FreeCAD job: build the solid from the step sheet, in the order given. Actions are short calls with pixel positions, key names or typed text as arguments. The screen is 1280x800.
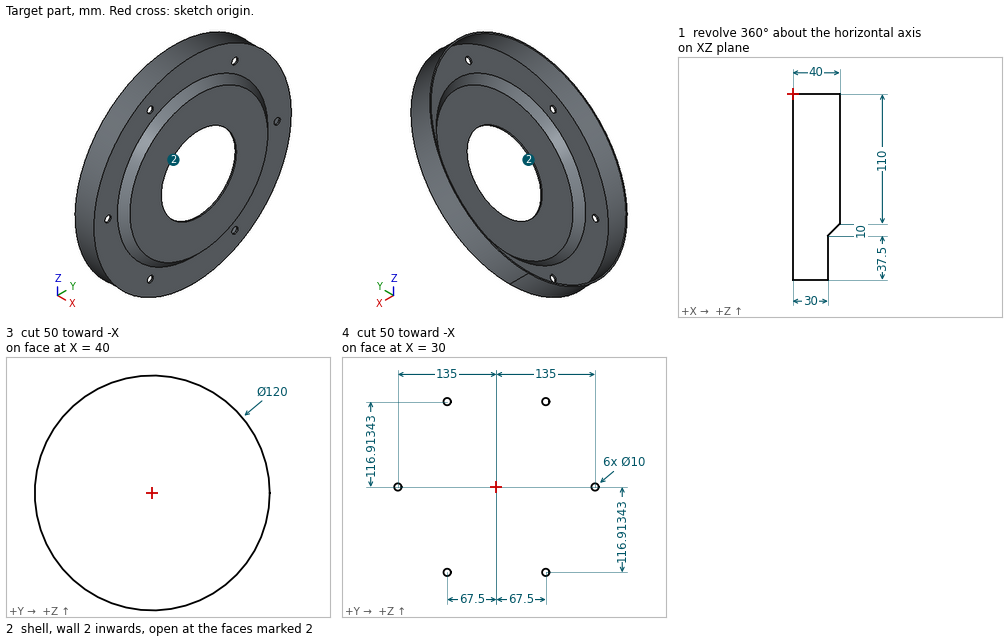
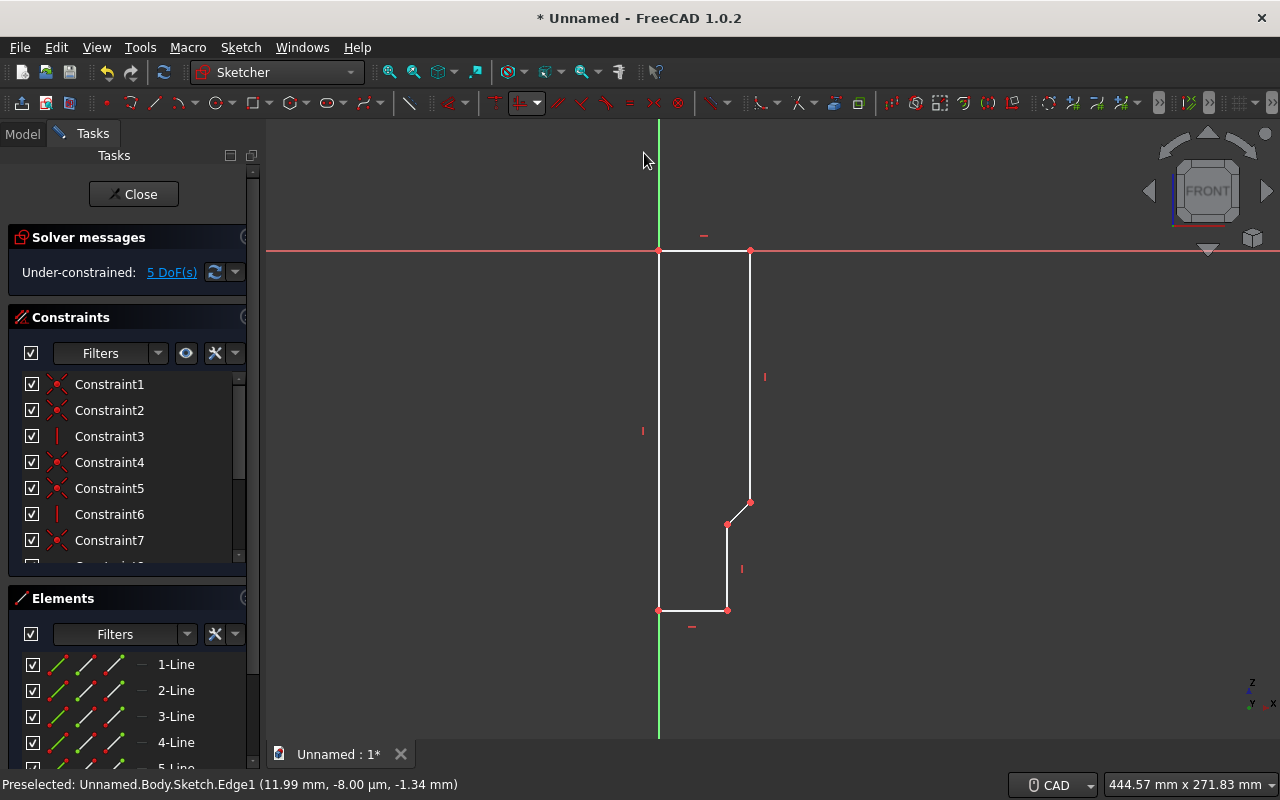
click(448, 104)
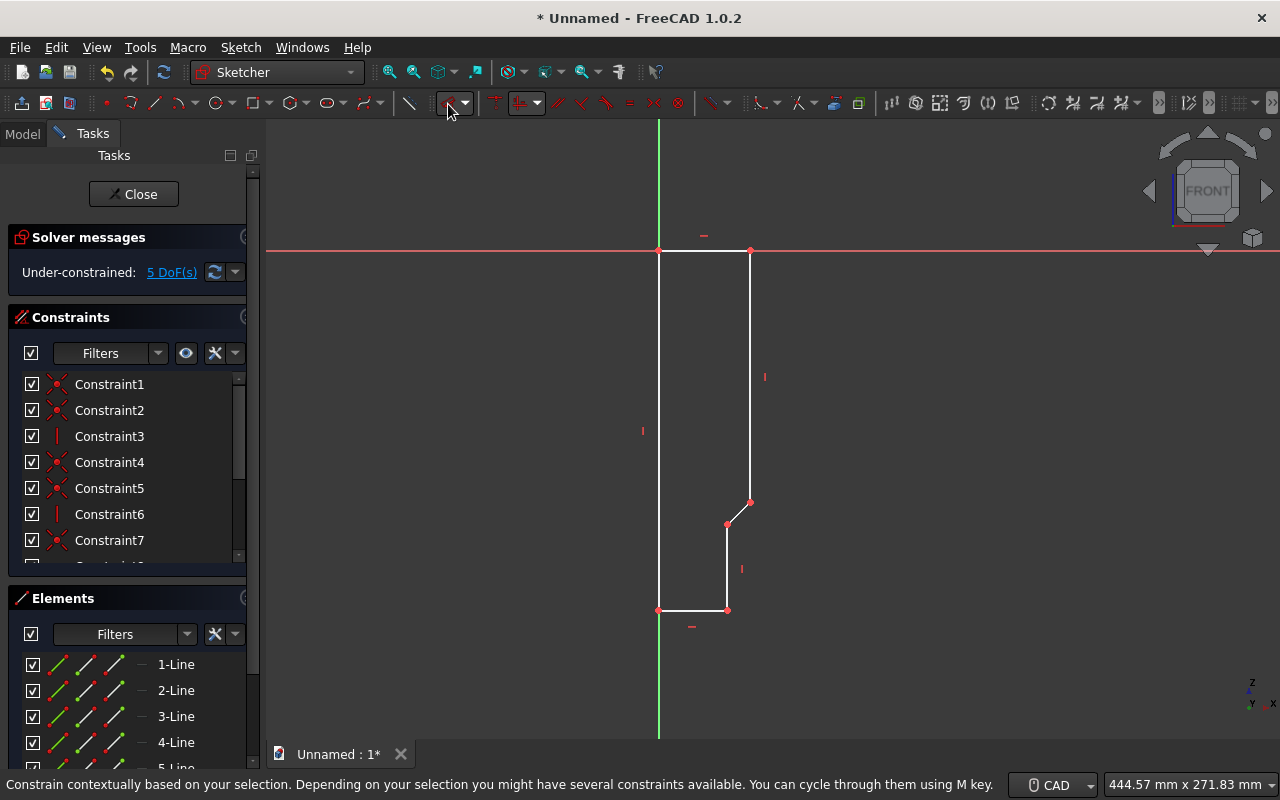
click(686, 251)
click(704, 217)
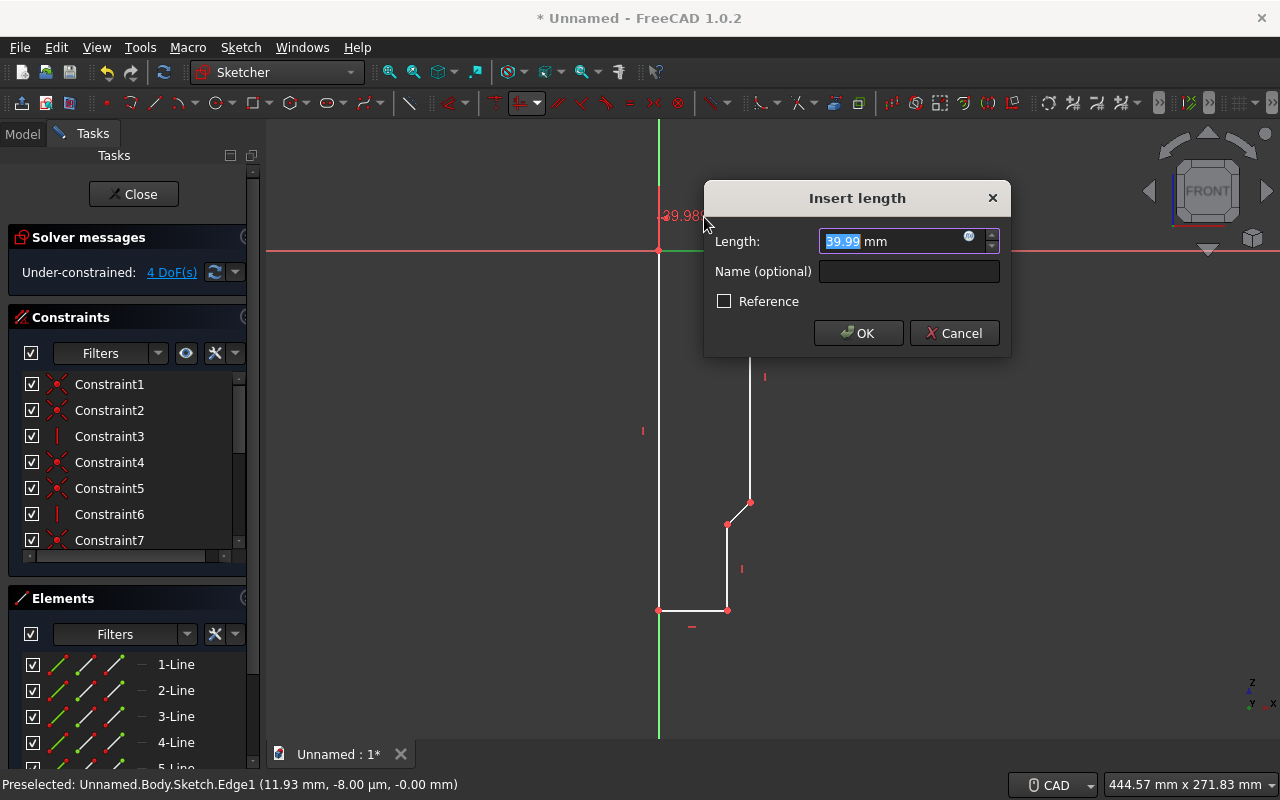
text(40)
key(Return)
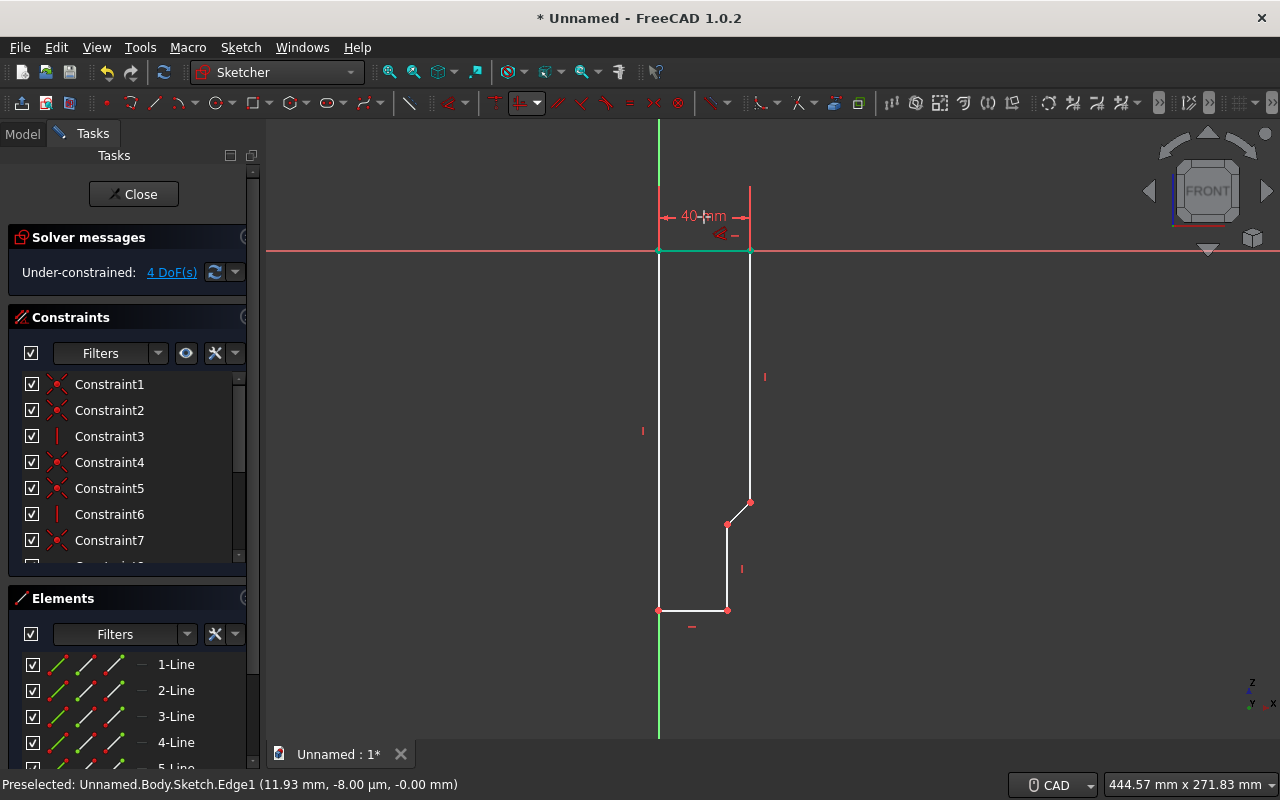
click(707, 611)
click(693, 645)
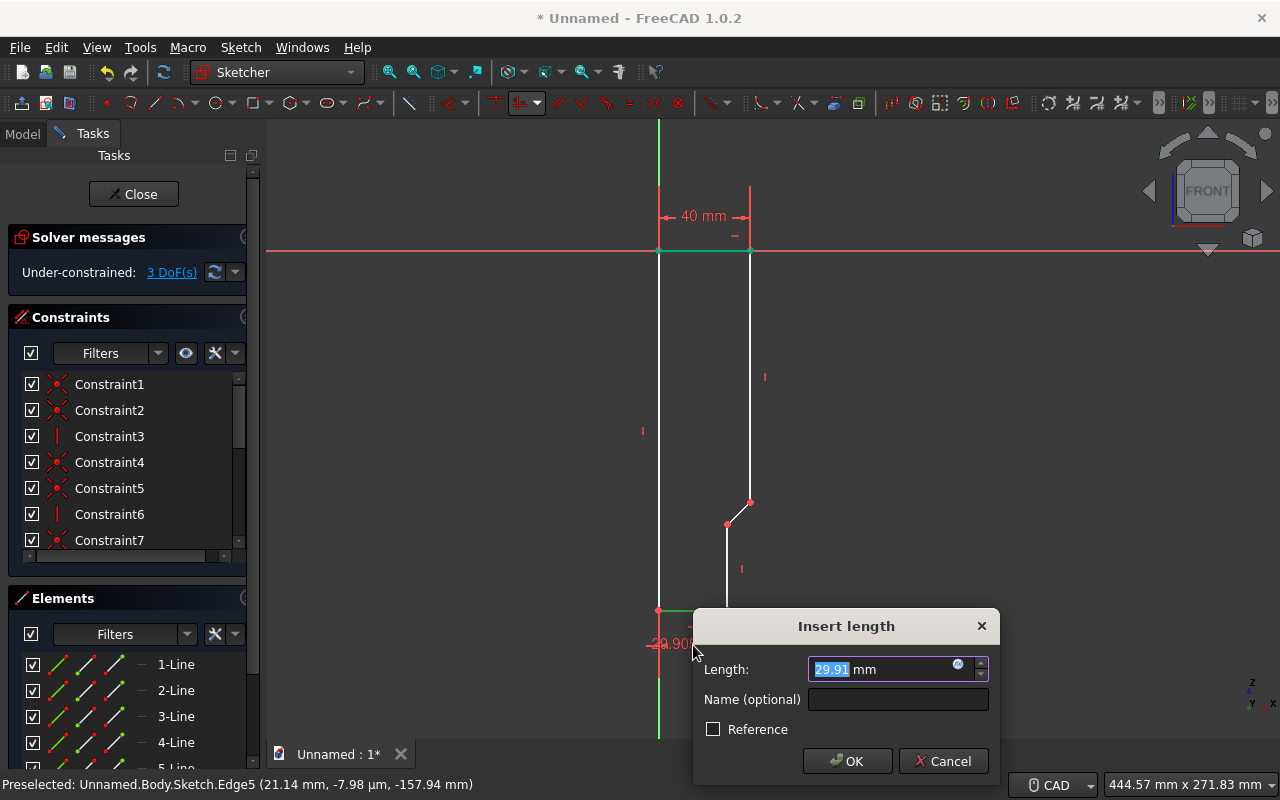
text(30)
key(Return)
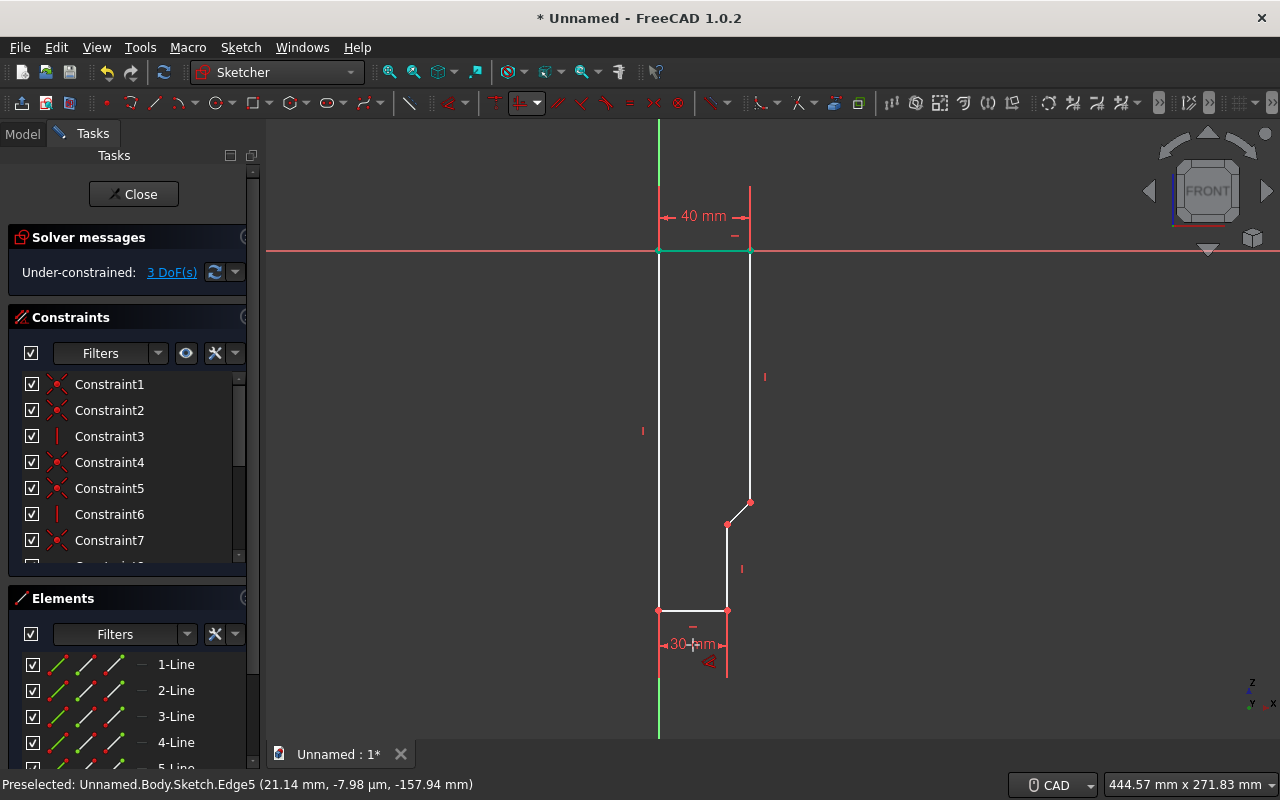
click(750, 326)
click(784, 377)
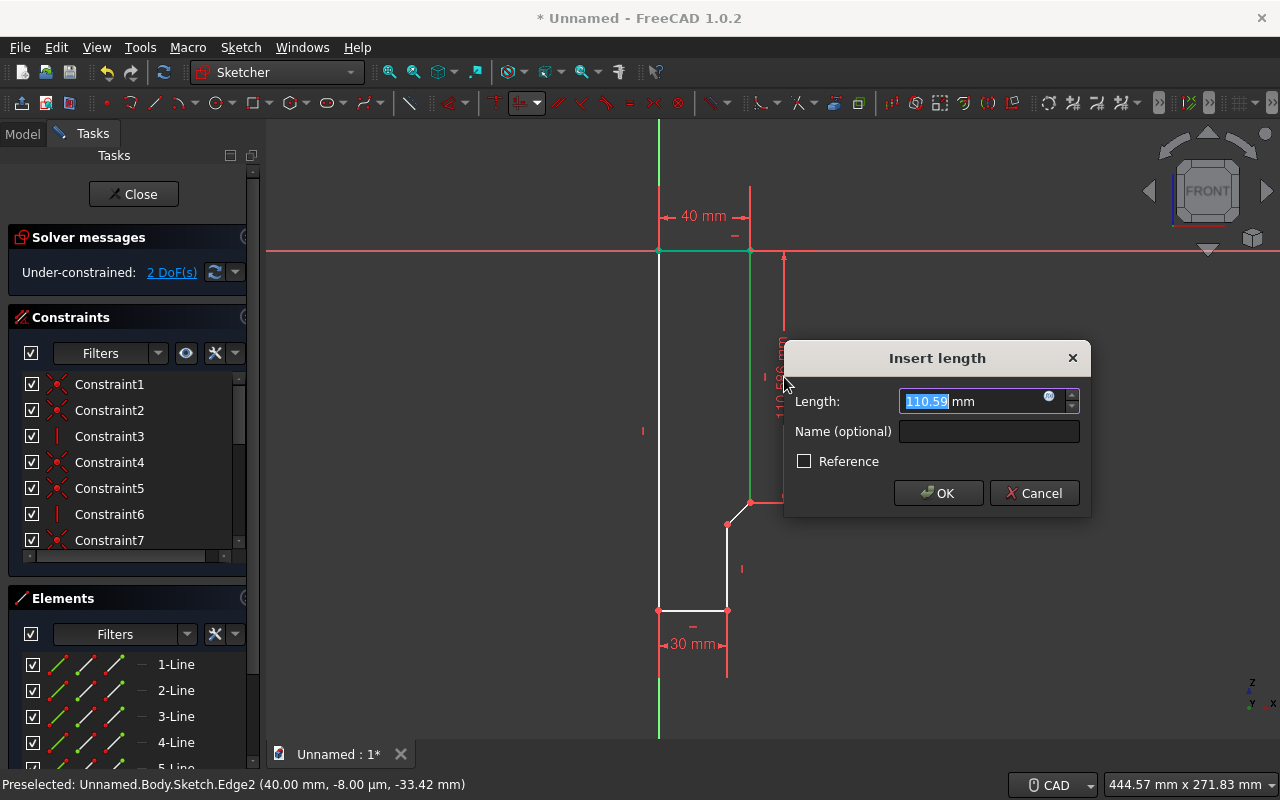
text(110)
key(Return)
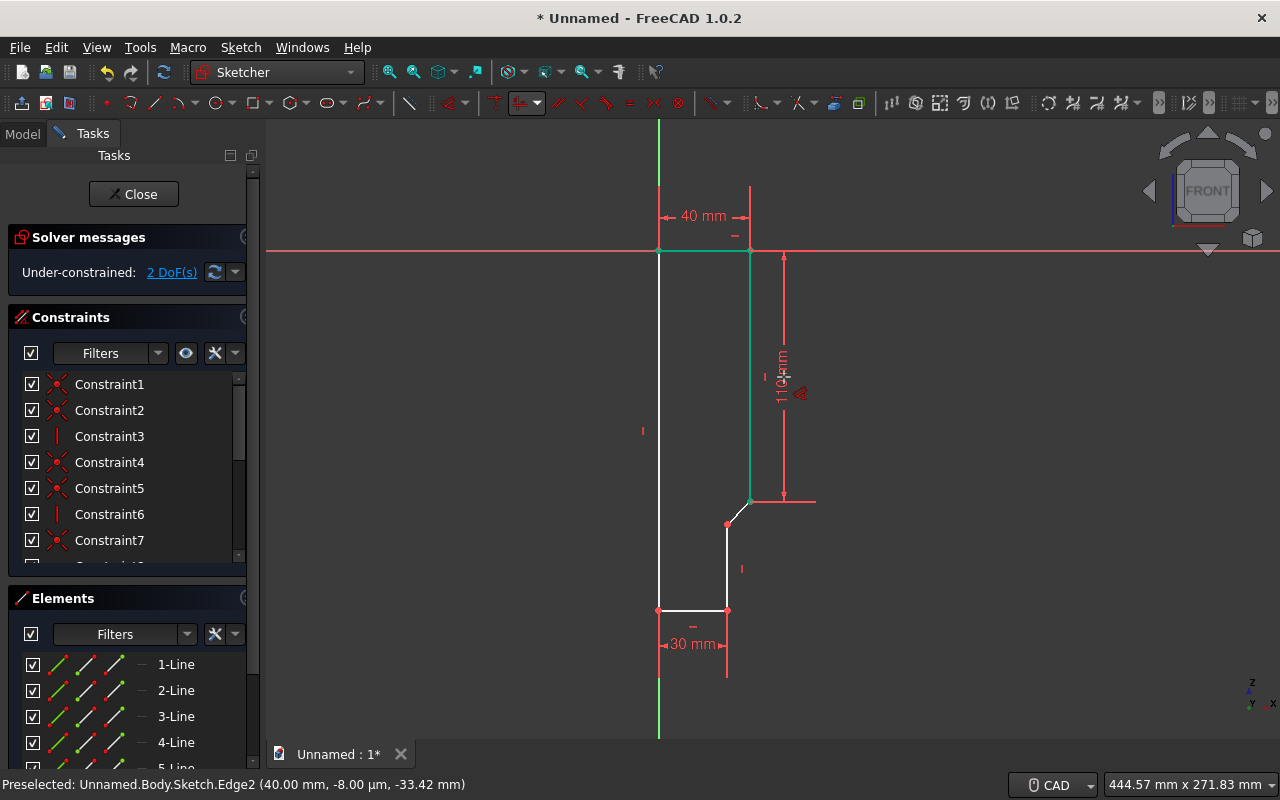
scroll(743, 509, up, 3)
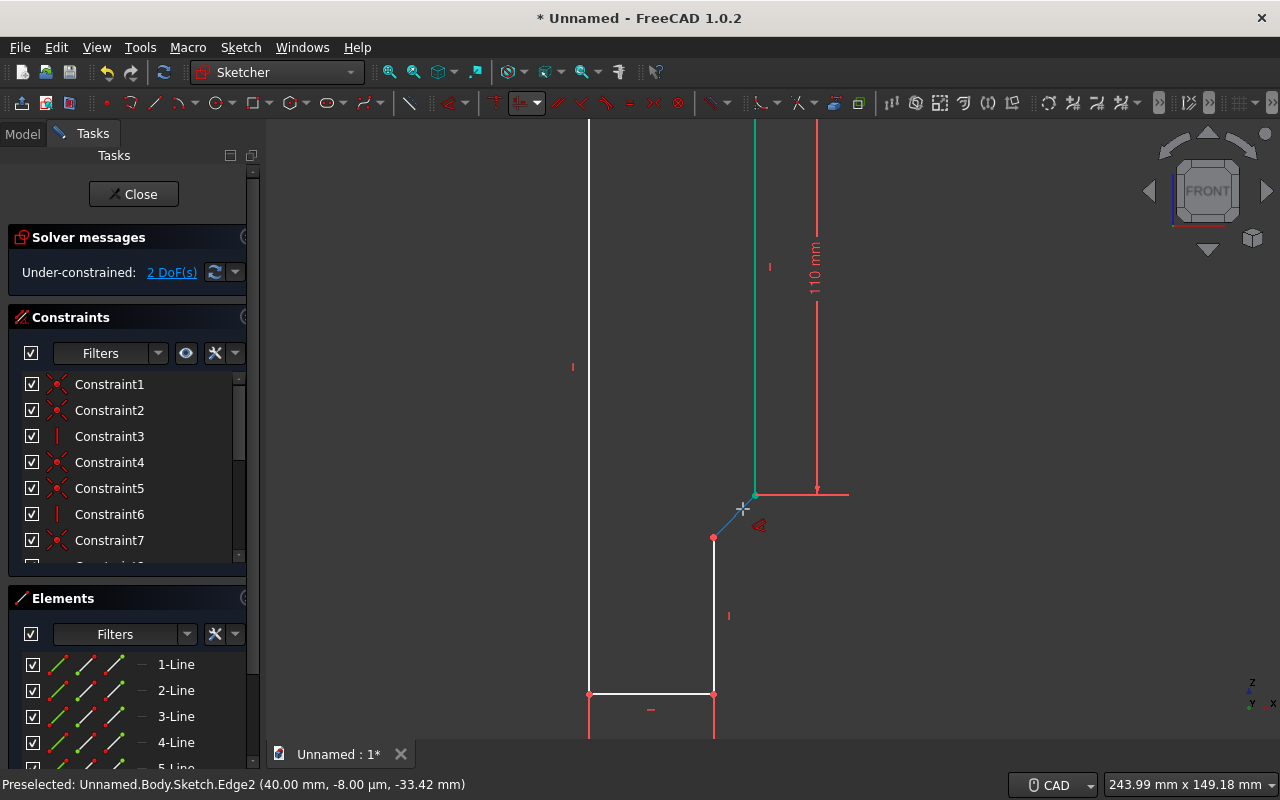
click(743, 508)
click(789, 516)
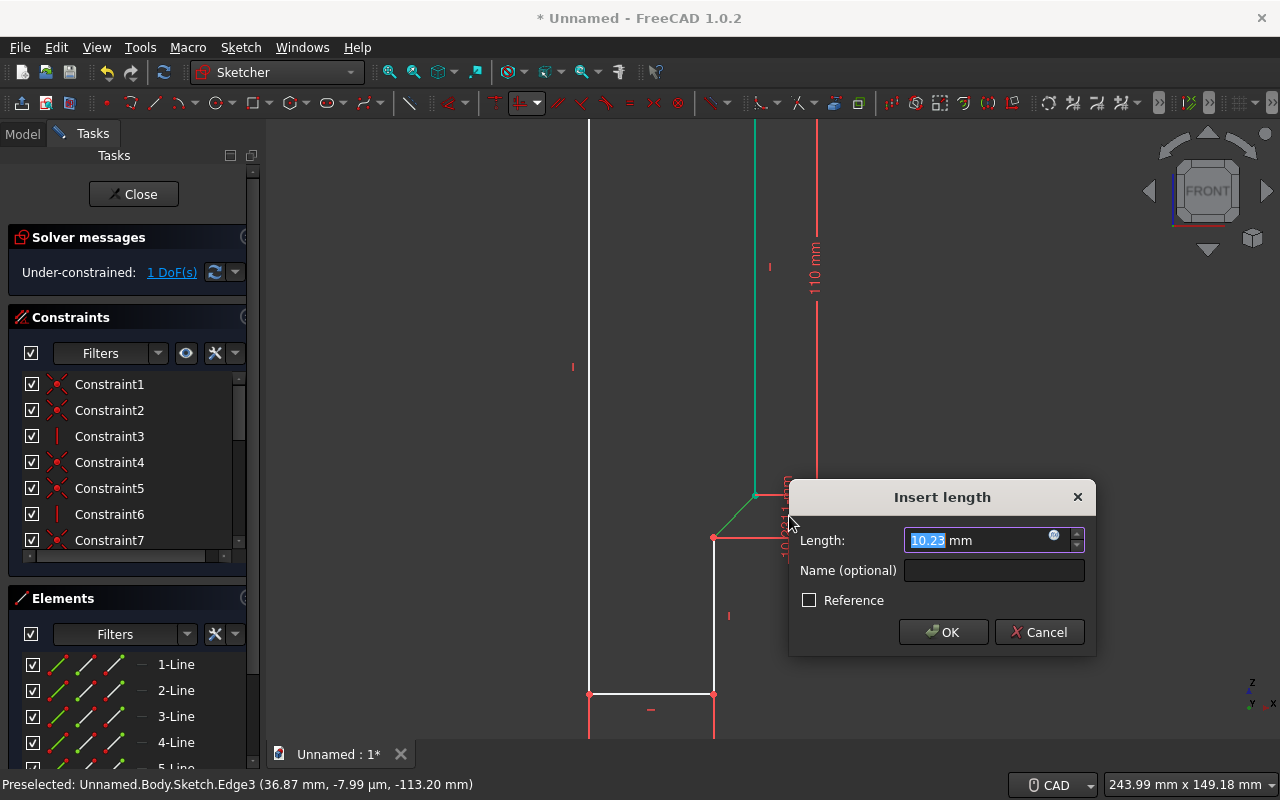
text(10)
key(Return)